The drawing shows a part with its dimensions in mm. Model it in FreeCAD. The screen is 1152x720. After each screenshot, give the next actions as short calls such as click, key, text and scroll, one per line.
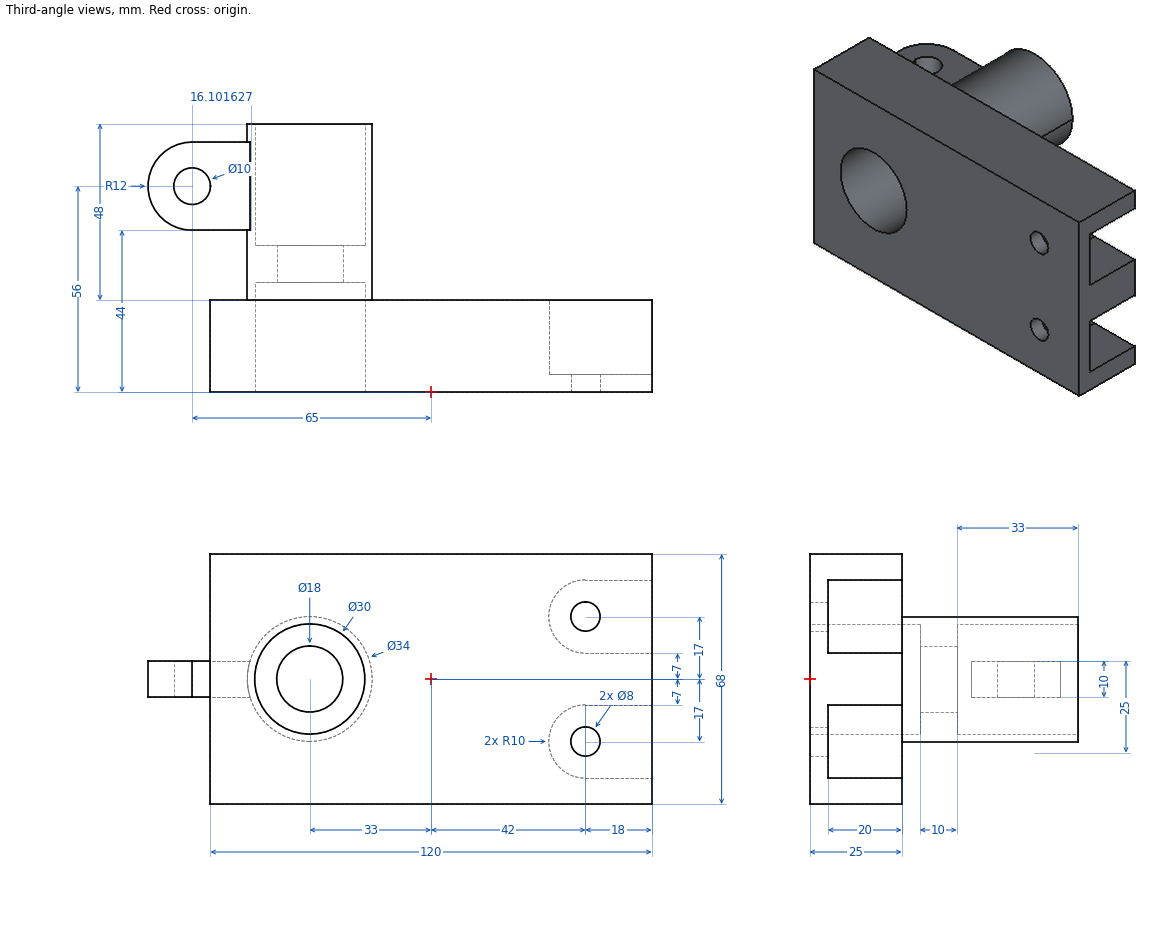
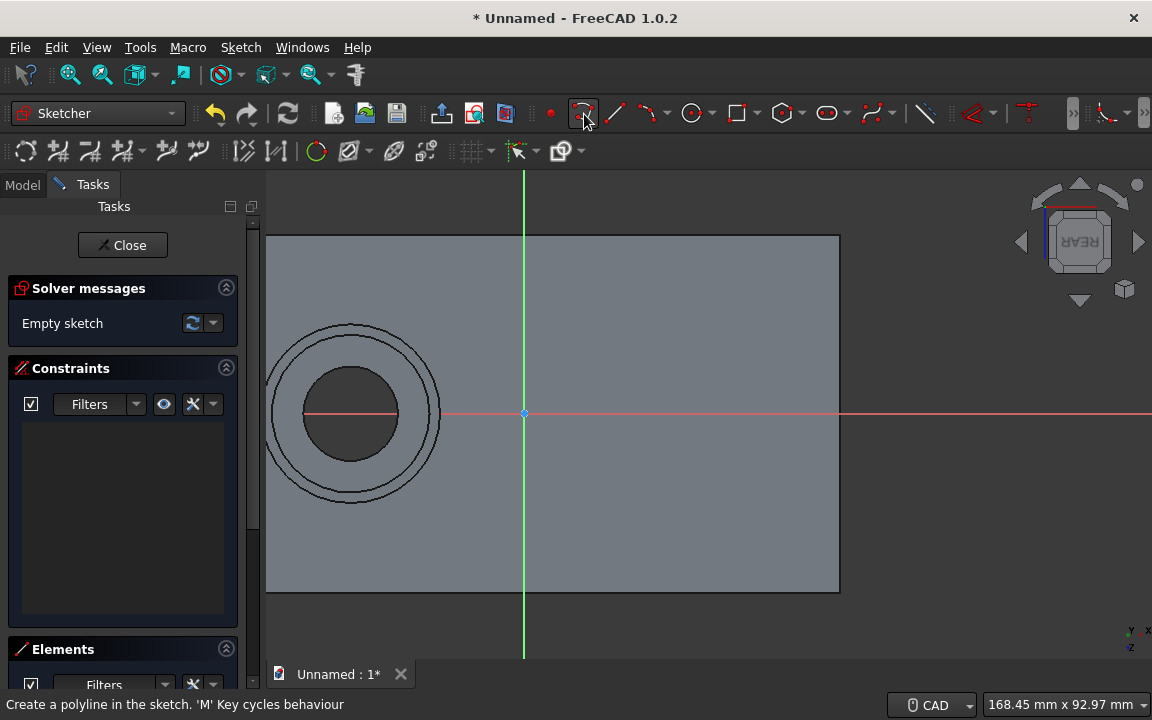
click(745, 377)
click(840, 377)
click(840, 272)
click(745, 272)
right_click(745, 272)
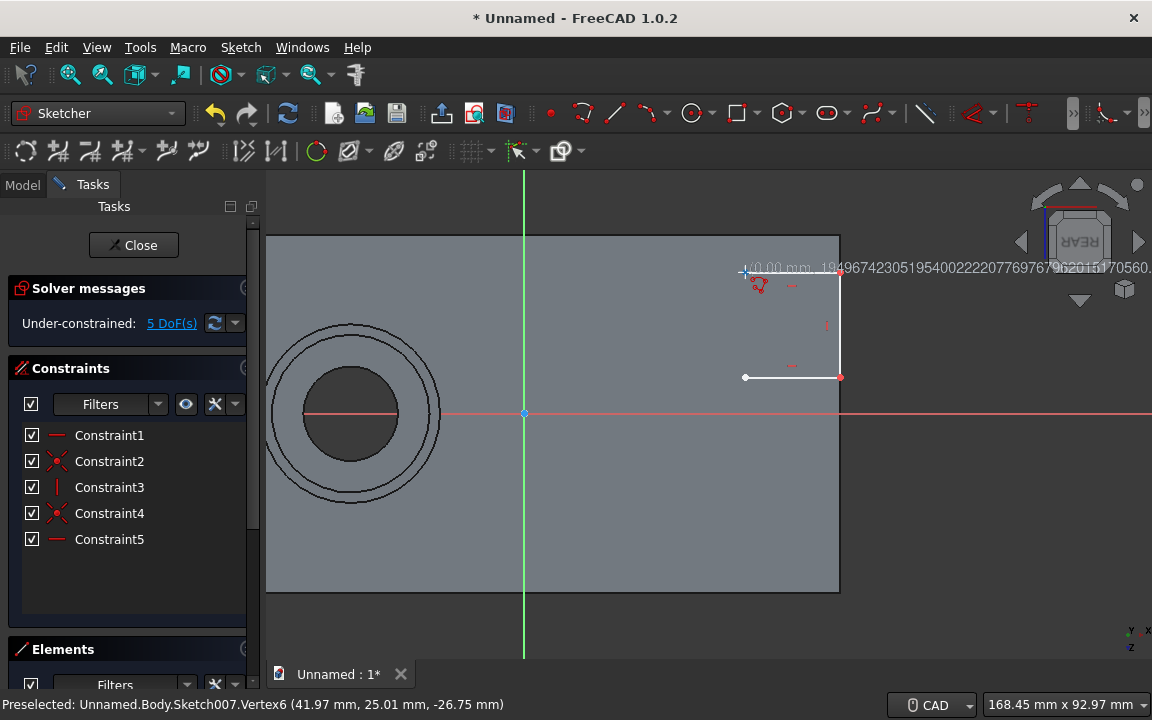
click(648, 114)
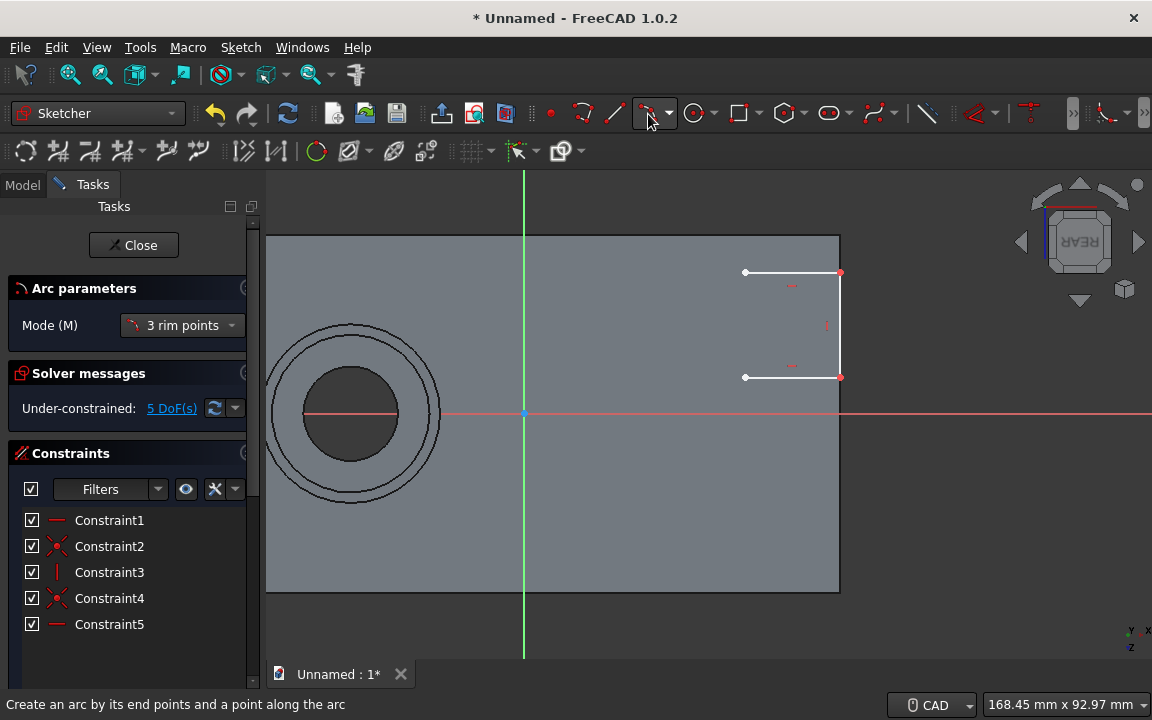
click(745, 273)
click(745, 378)
click(693, 324)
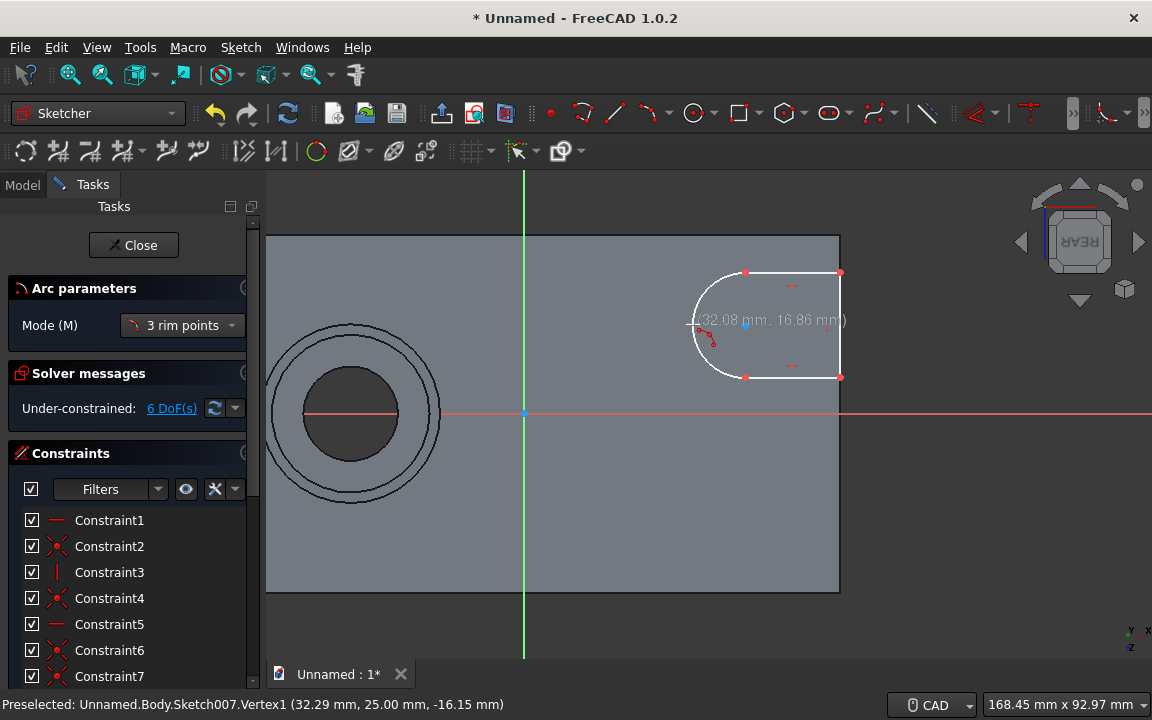
click(584, 114)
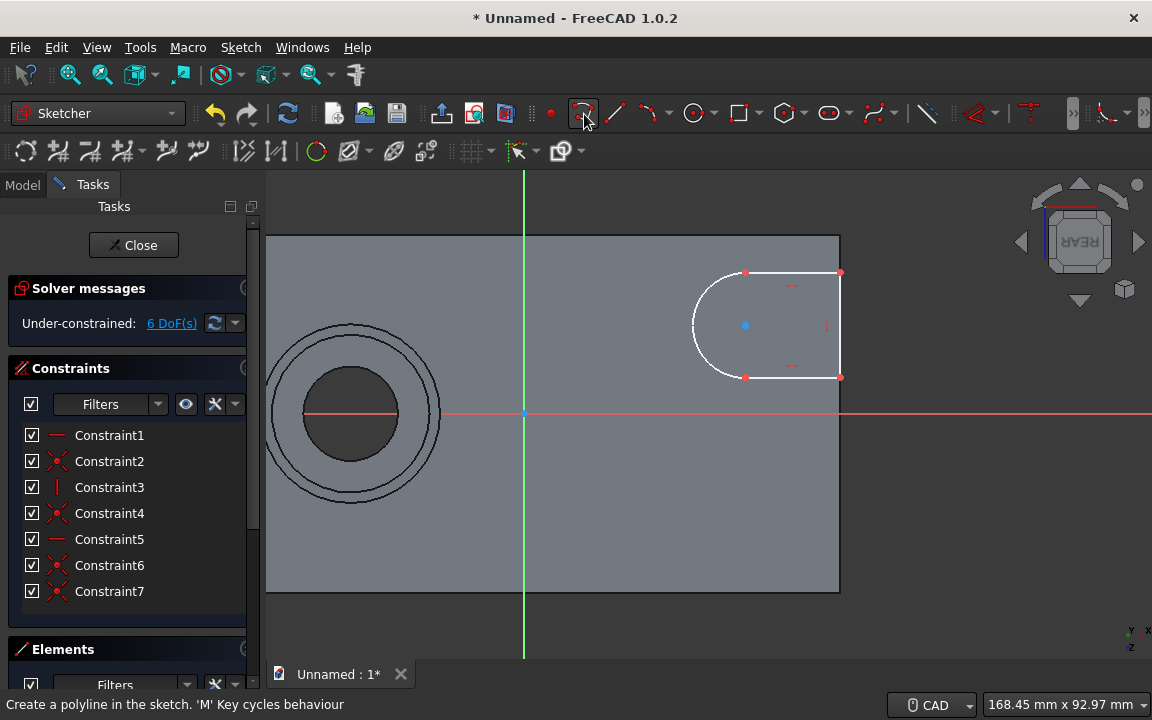
click(745, 556)
click(840, 556)
click(840, 450)
click(745, 450)
right_click(745, 450)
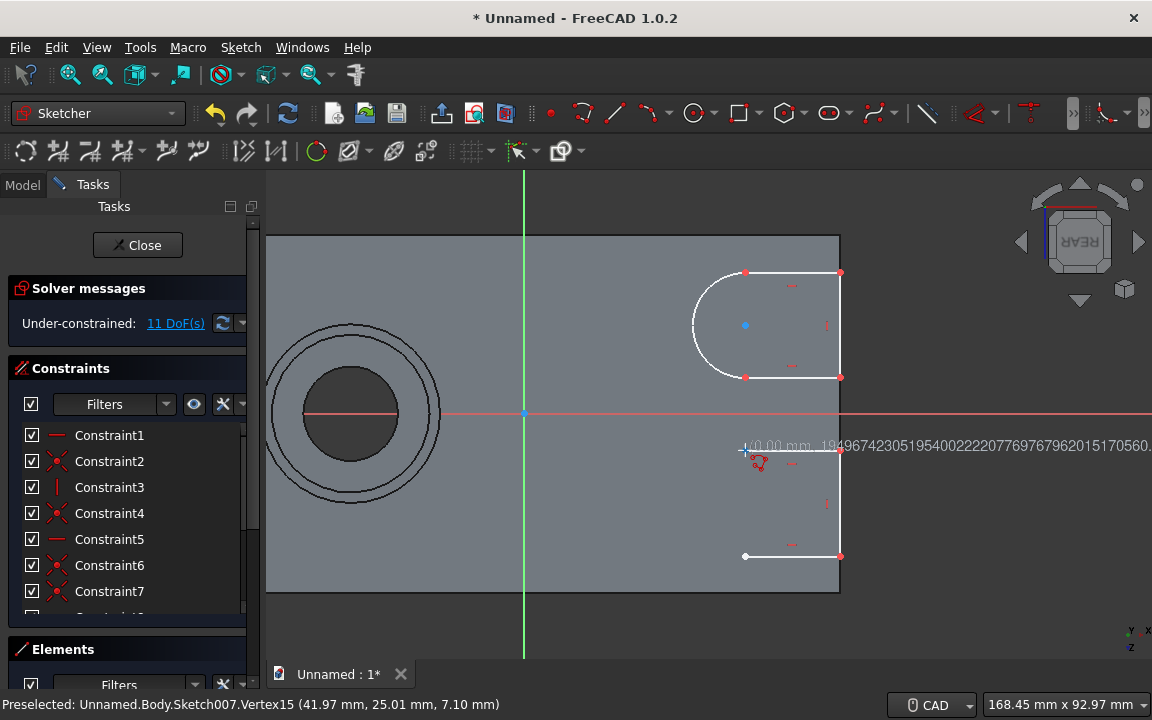
click(648, 114)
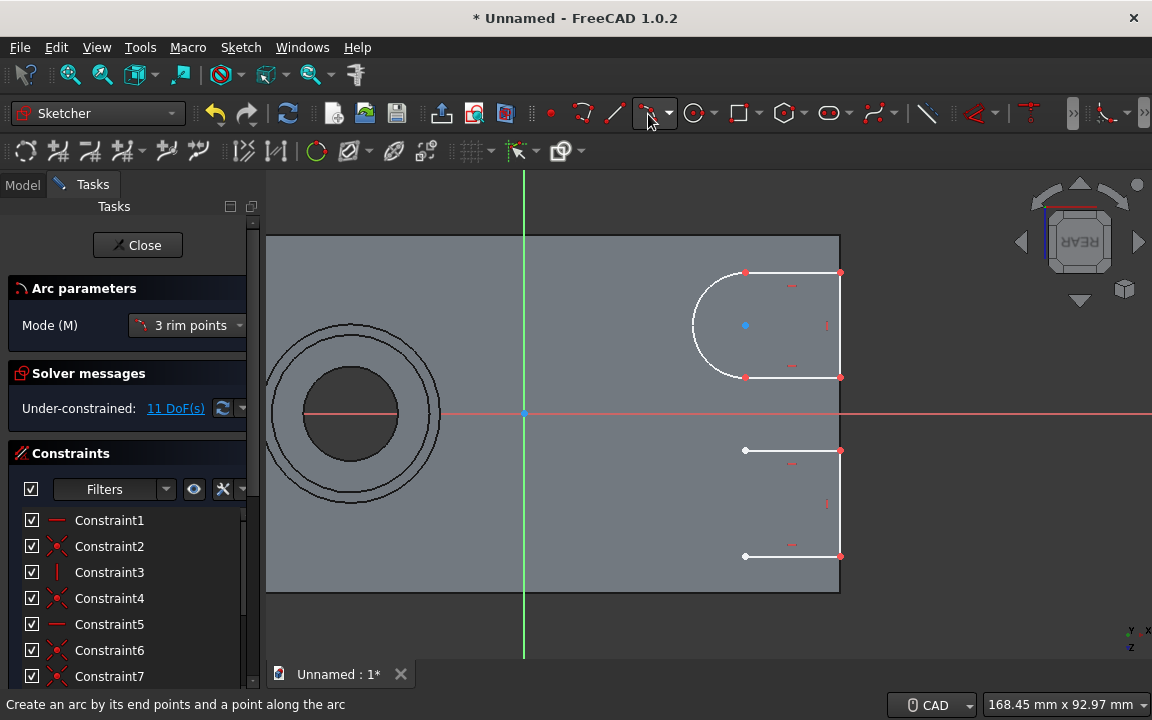
click(745, 451)
click(745, 557)
click(693, 503)
key(Escape)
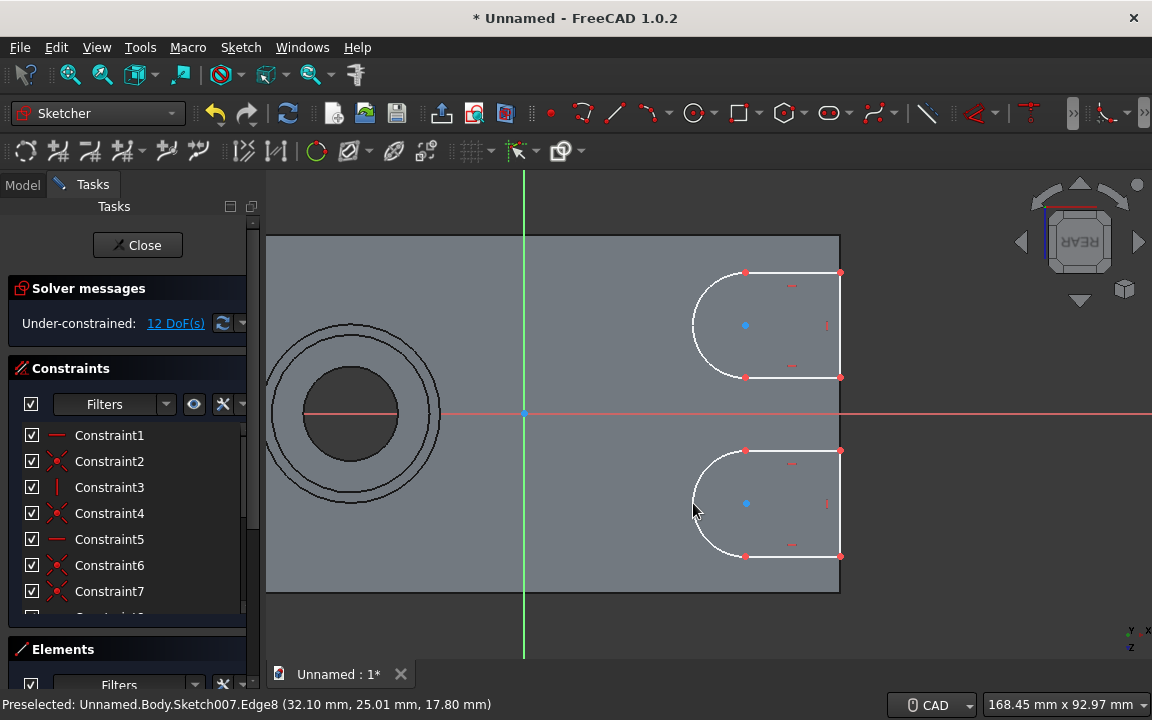
click(774, 378)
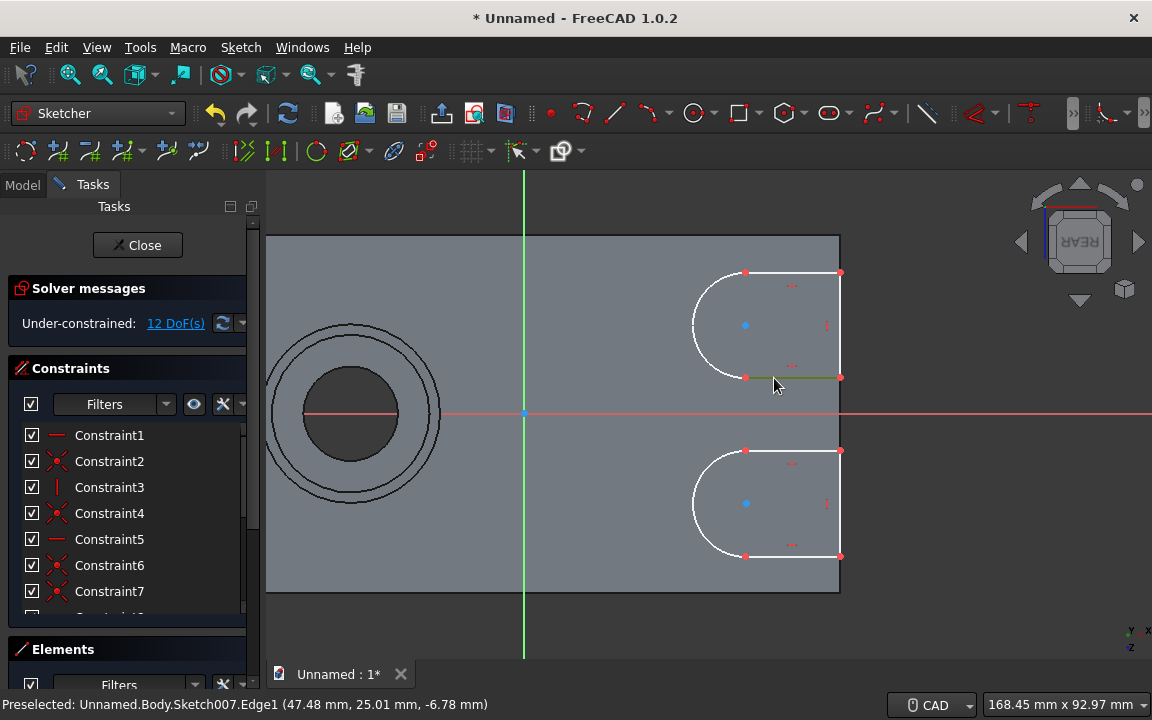
click(703, 295)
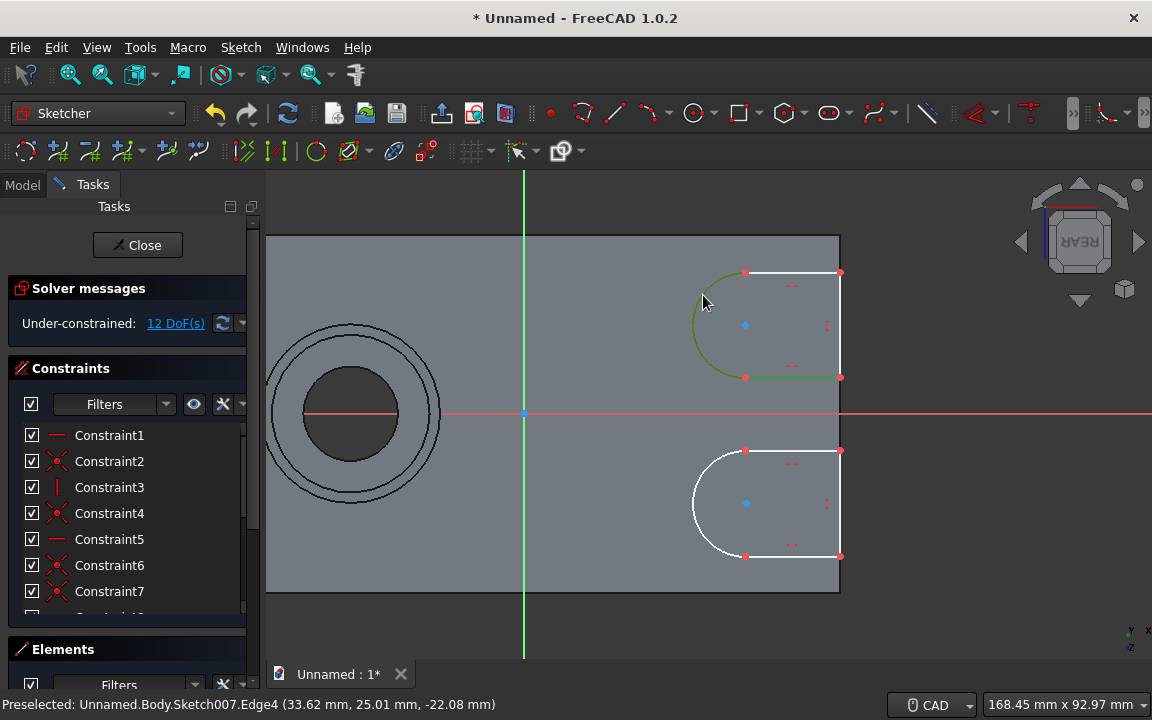
key(t)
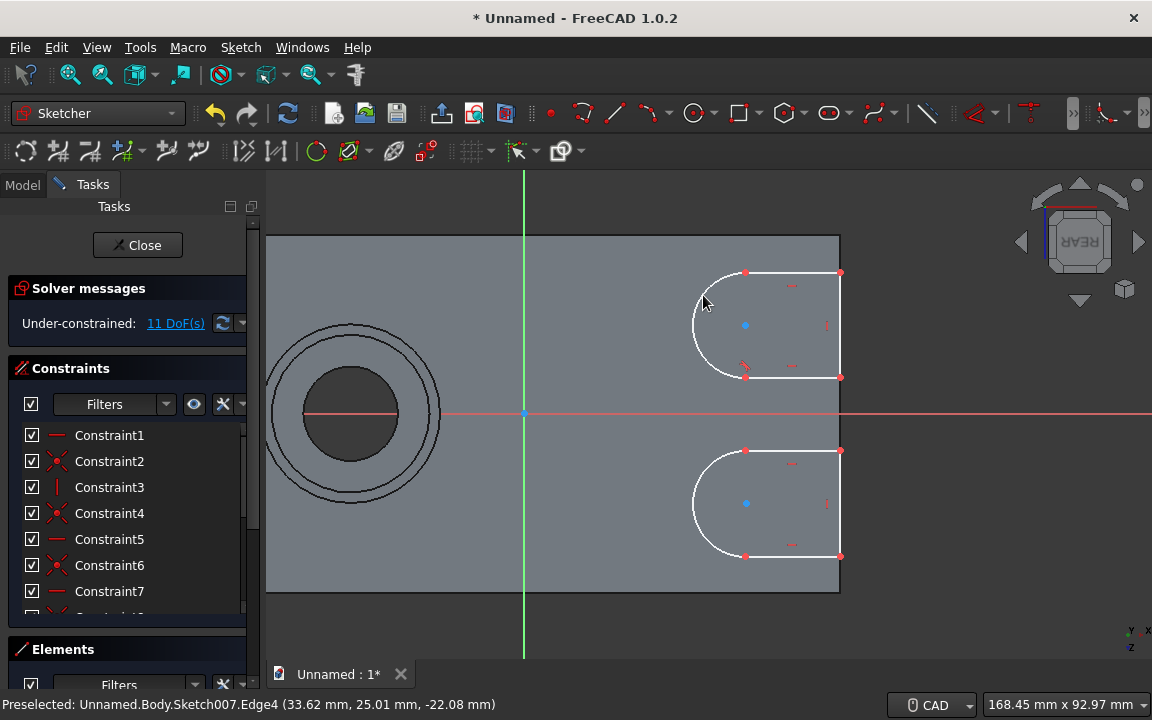
click(812, 273)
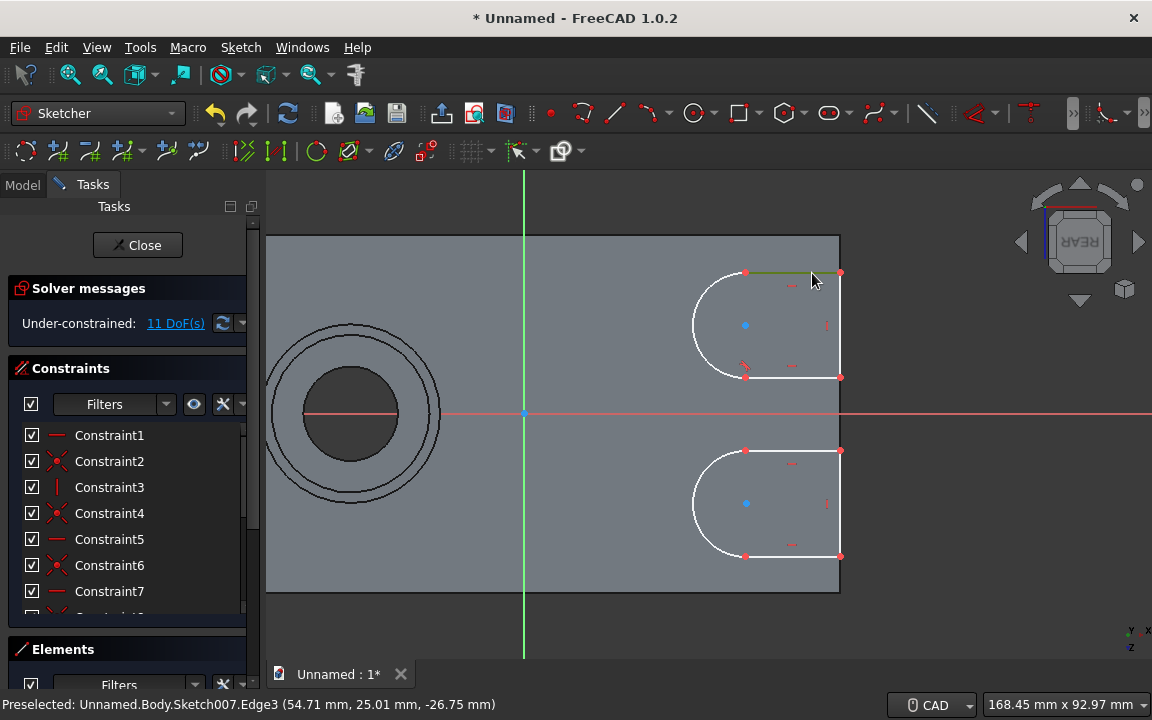
click(703, 295)